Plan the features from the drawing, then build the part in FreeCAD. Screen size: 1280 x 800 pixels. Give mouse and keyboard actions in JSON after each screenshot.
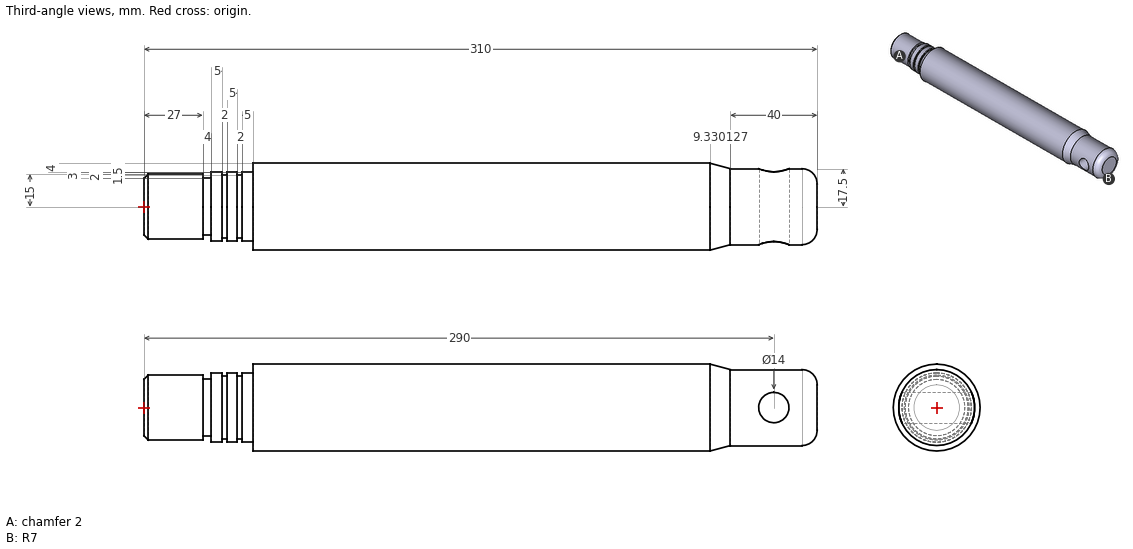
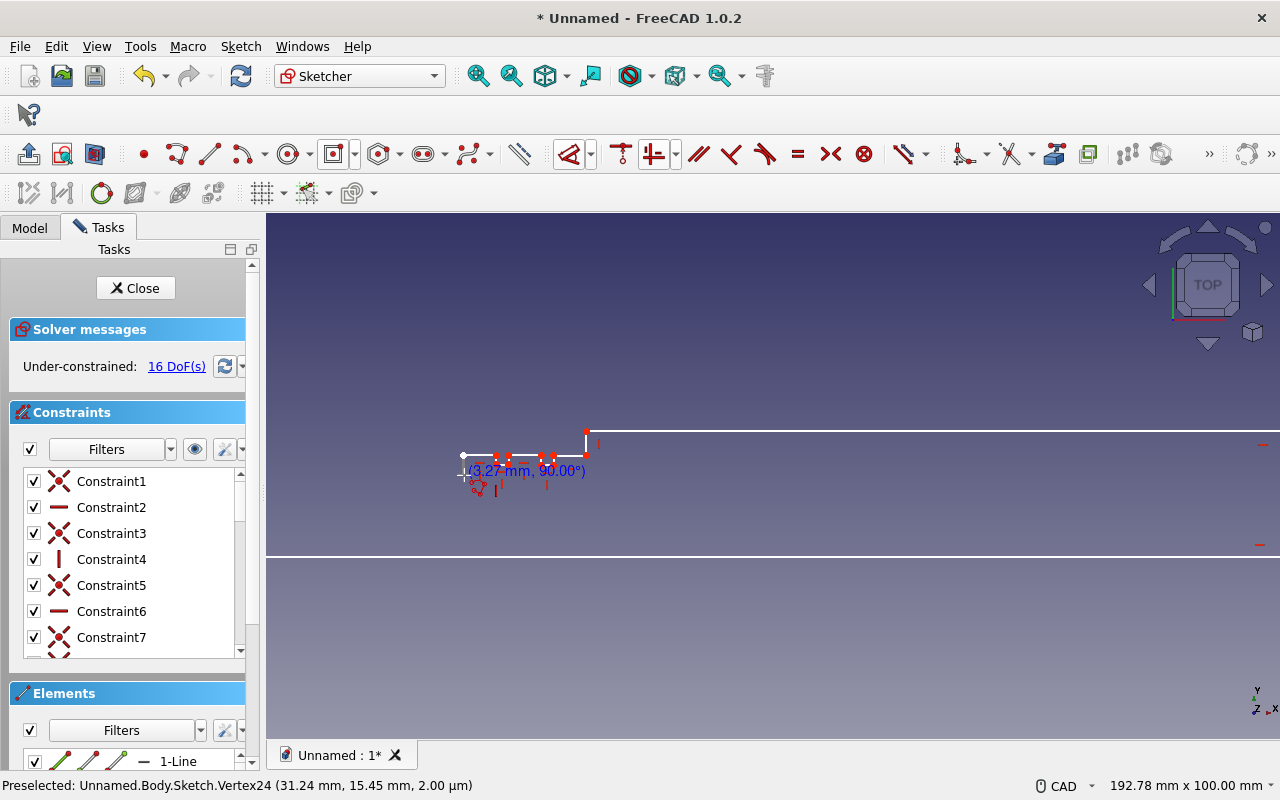
{"action": "left_click", "coordinate": [464, 474]}
{"action": "left_click", "coordinate": [438, 474]}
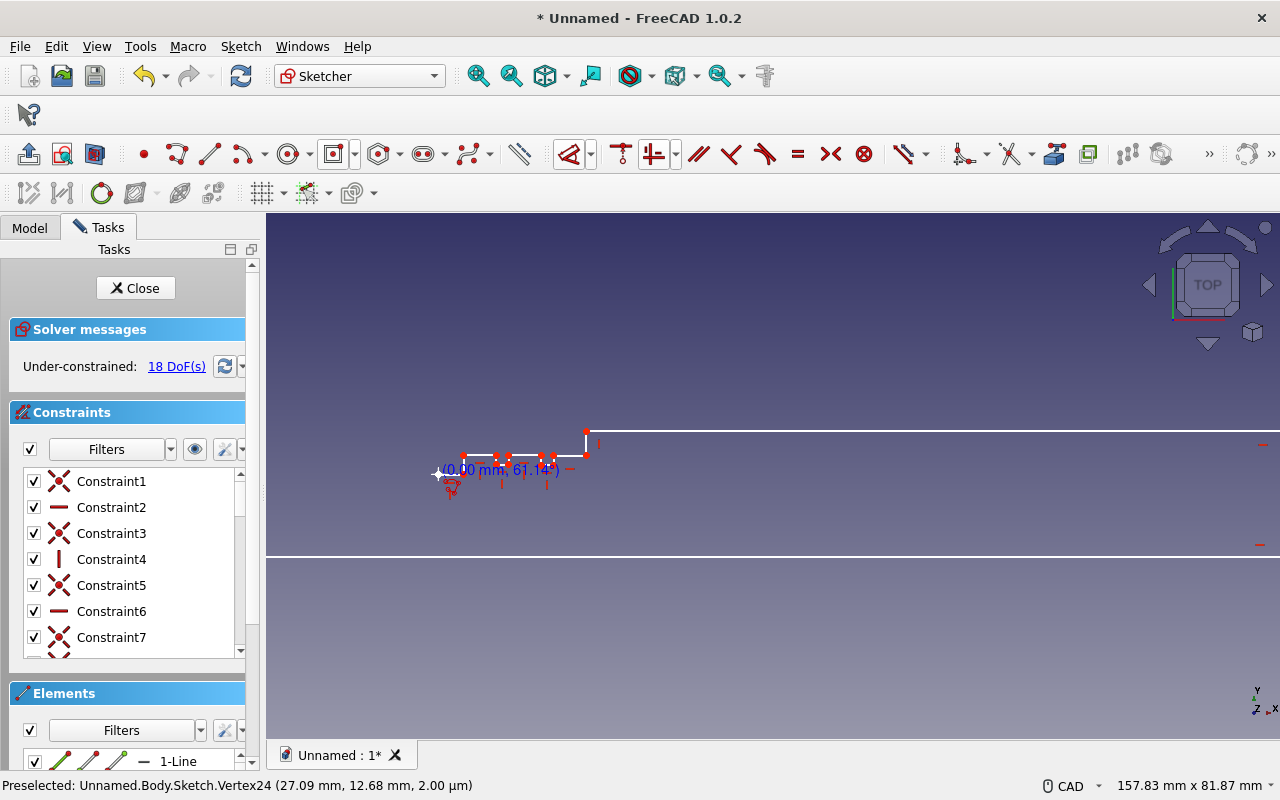
{"action": "scroll", "coordinate": [438, 461], "scroll_direction": "up", "scroll_amount": 2}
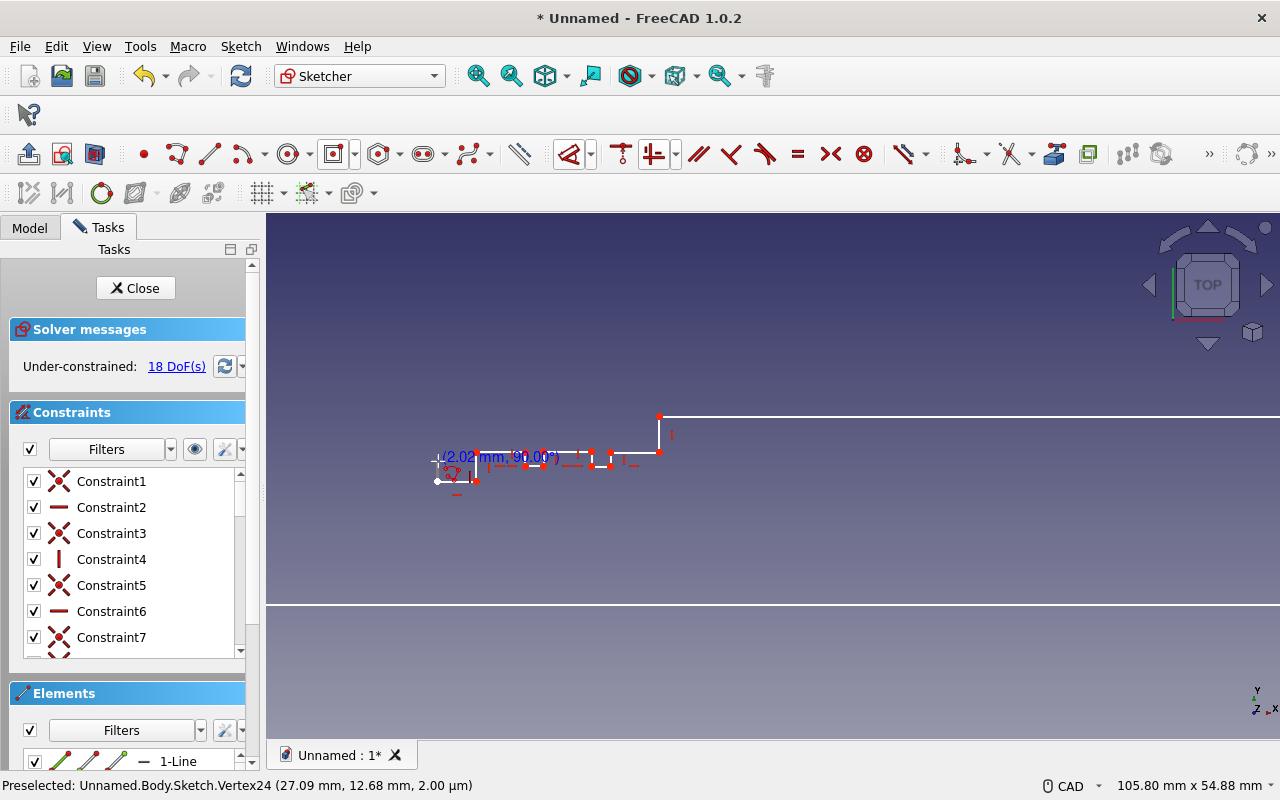
{"action": "left_click", "coordinate": [438, 461]}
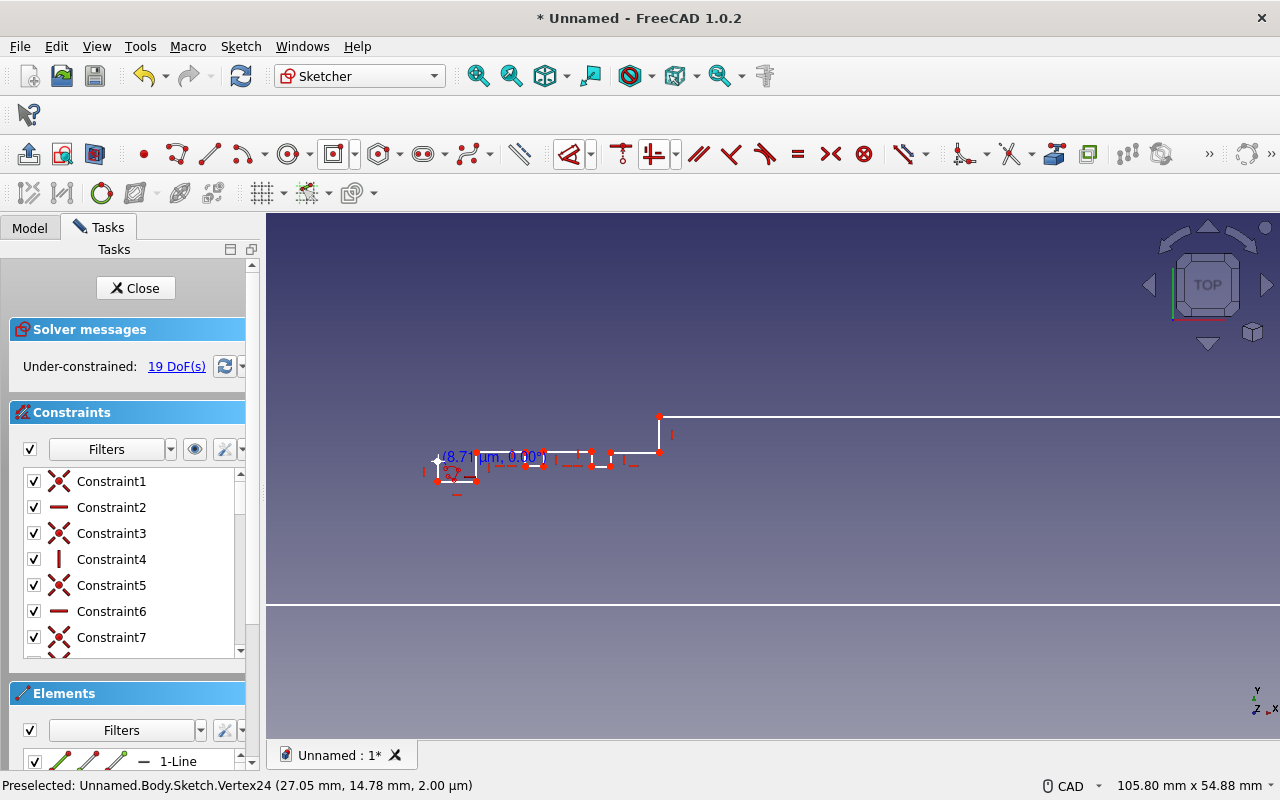
{"action": "scroll", "coordinate": [461, 468], "scroll_direction": "down", "scroll_amount": 8}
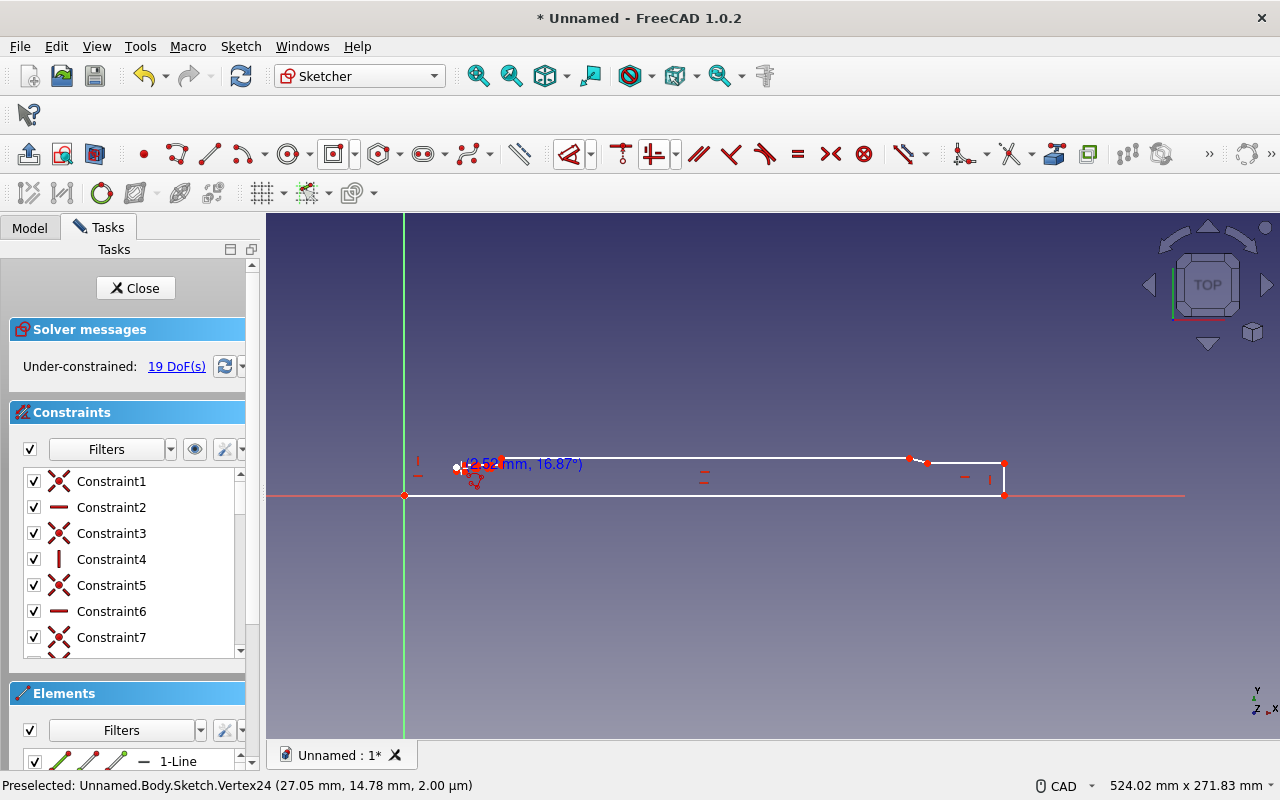
{"action": "left_click", "coordinate": [413, 467]}
{"action": "left_click", "coordinate": [404, 496]}
{"action": "key", "text": "Escape"}
{"action": "key", "text": "Escape"}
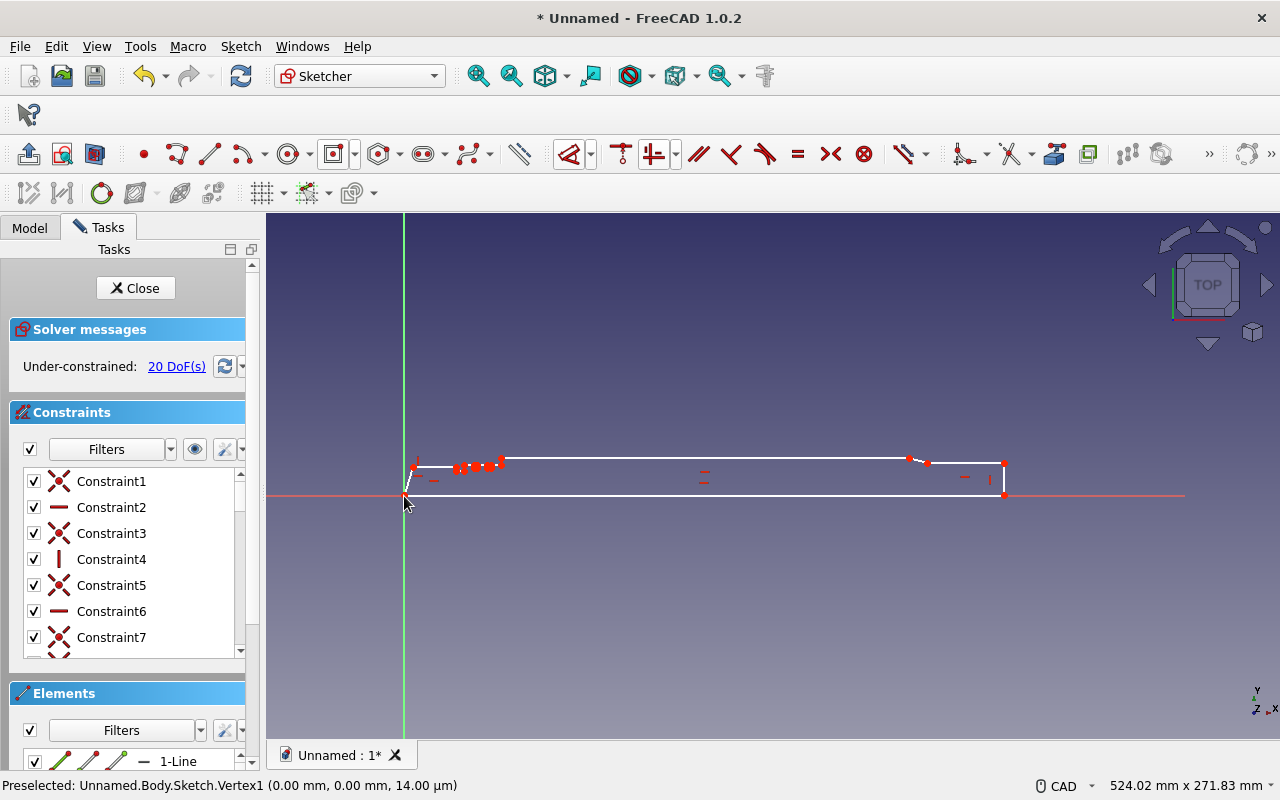
{"action": "left_click", "coordinate": [408, 484]}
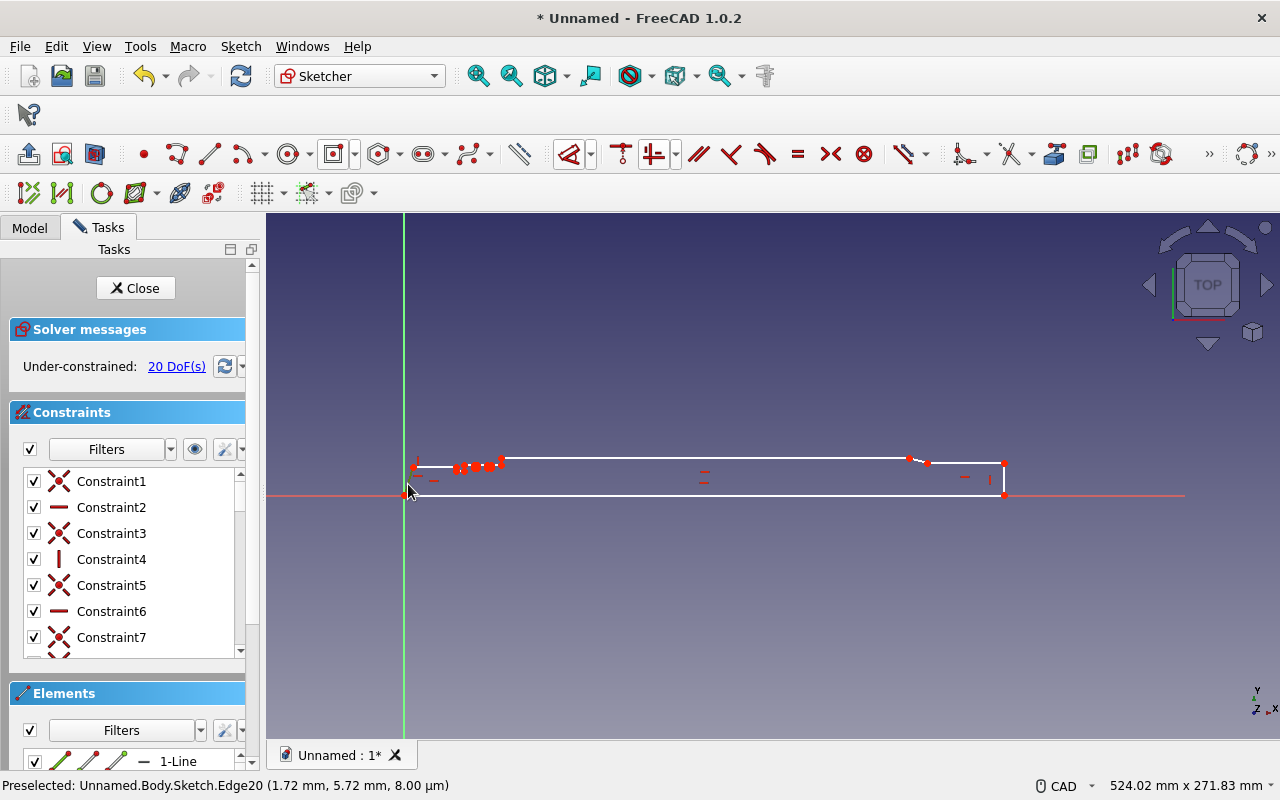
{"action": "left_click", "coordinate": [676, 154]}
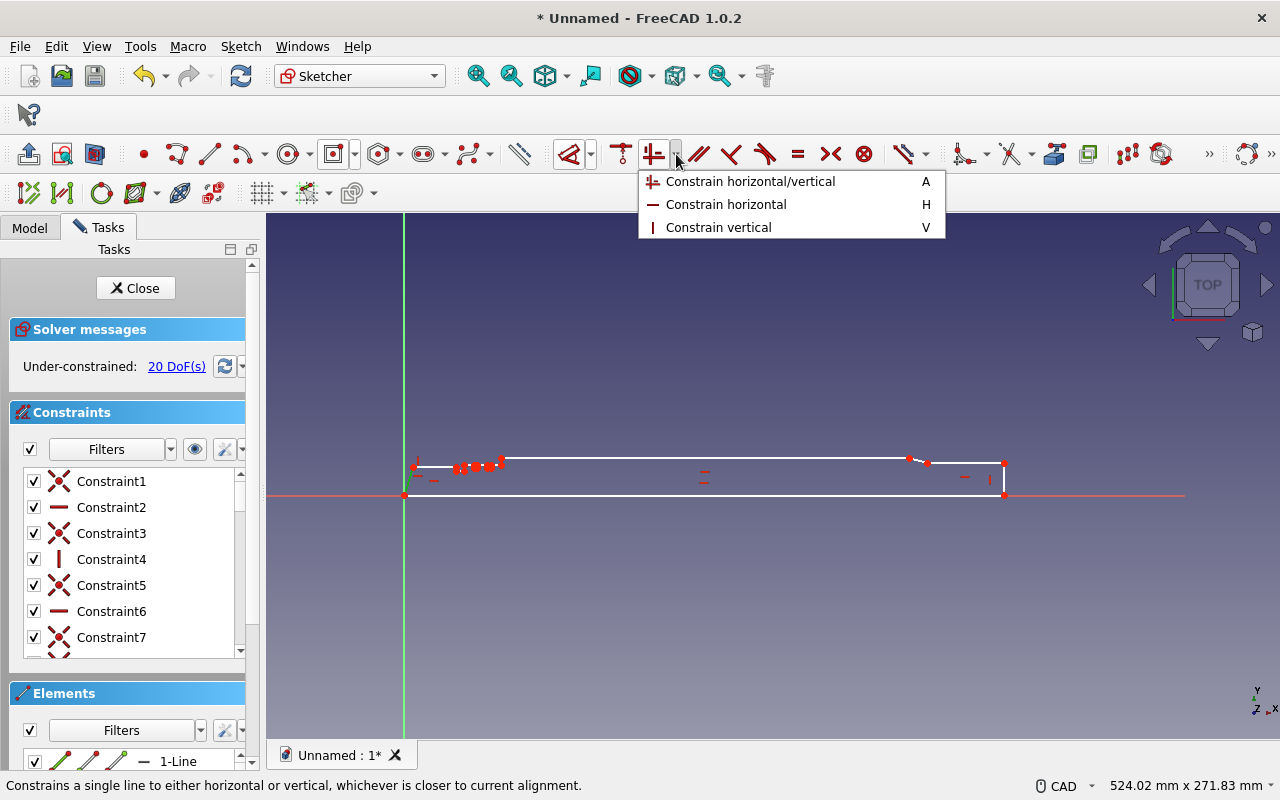
{"action": "left_click", "coordinate": [792, 228]}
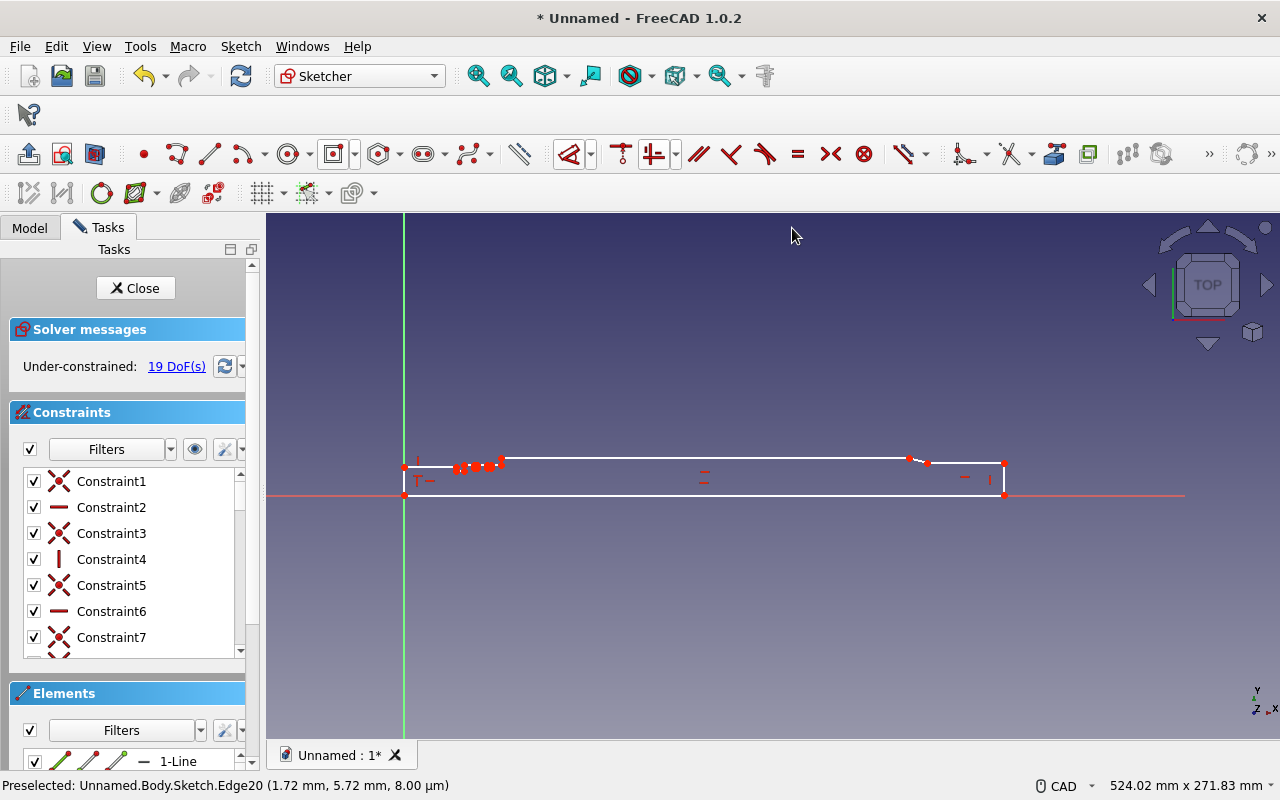
{"action": "scroll", "coordinate": [501, 462], "scroll_direction": "up", "scroll_amount": 9}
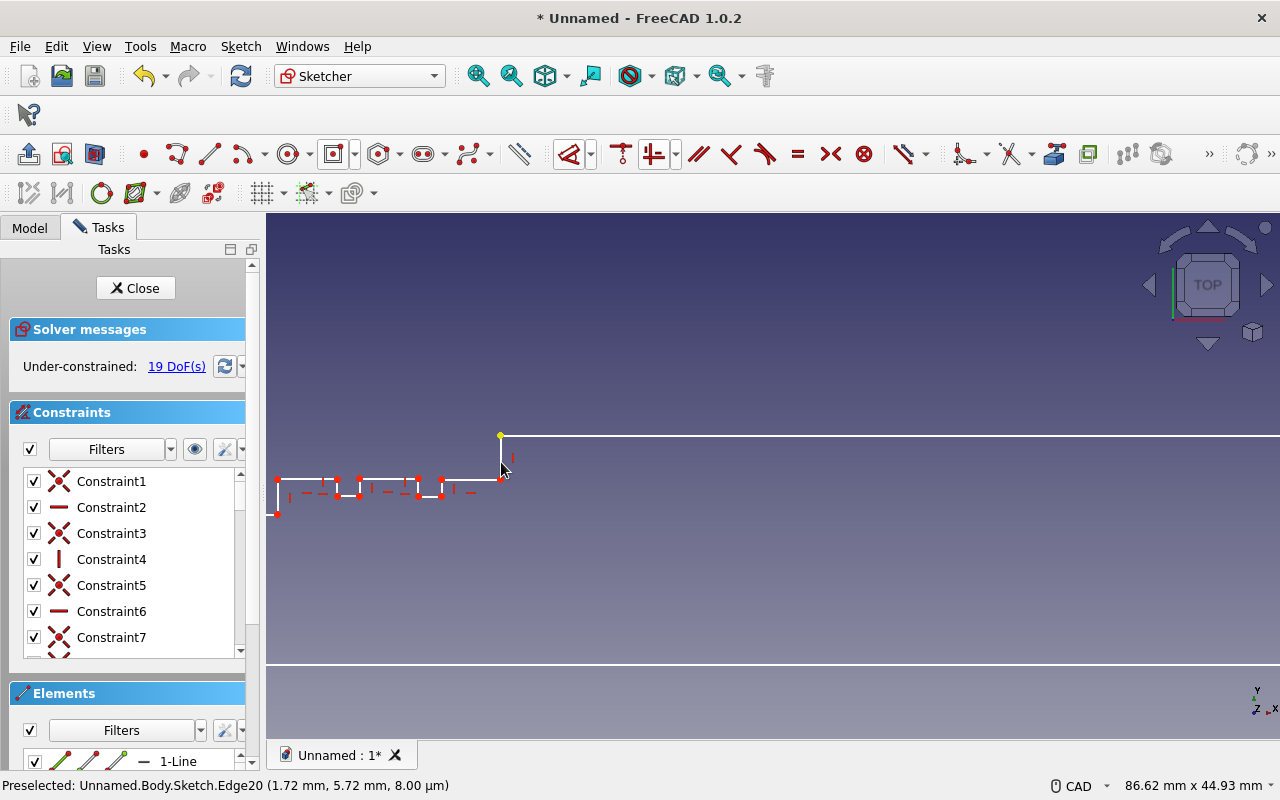
{"action": "left_click", "coordinate": [501, 458]}